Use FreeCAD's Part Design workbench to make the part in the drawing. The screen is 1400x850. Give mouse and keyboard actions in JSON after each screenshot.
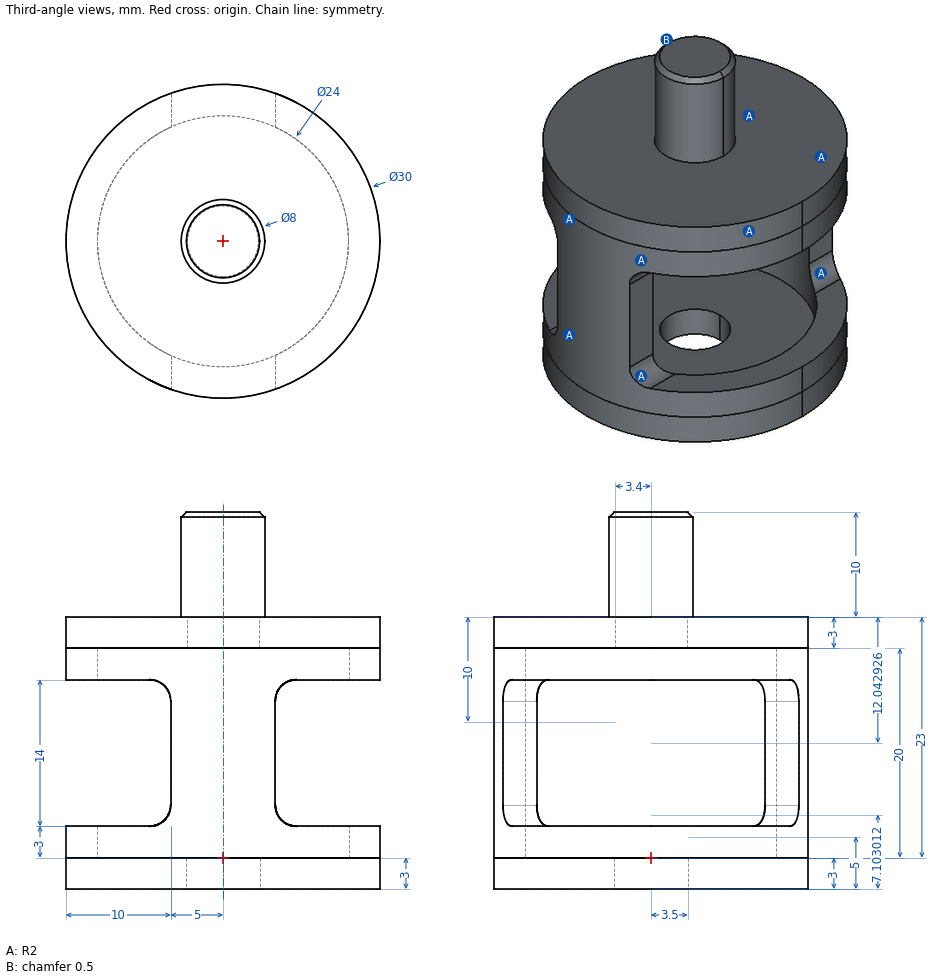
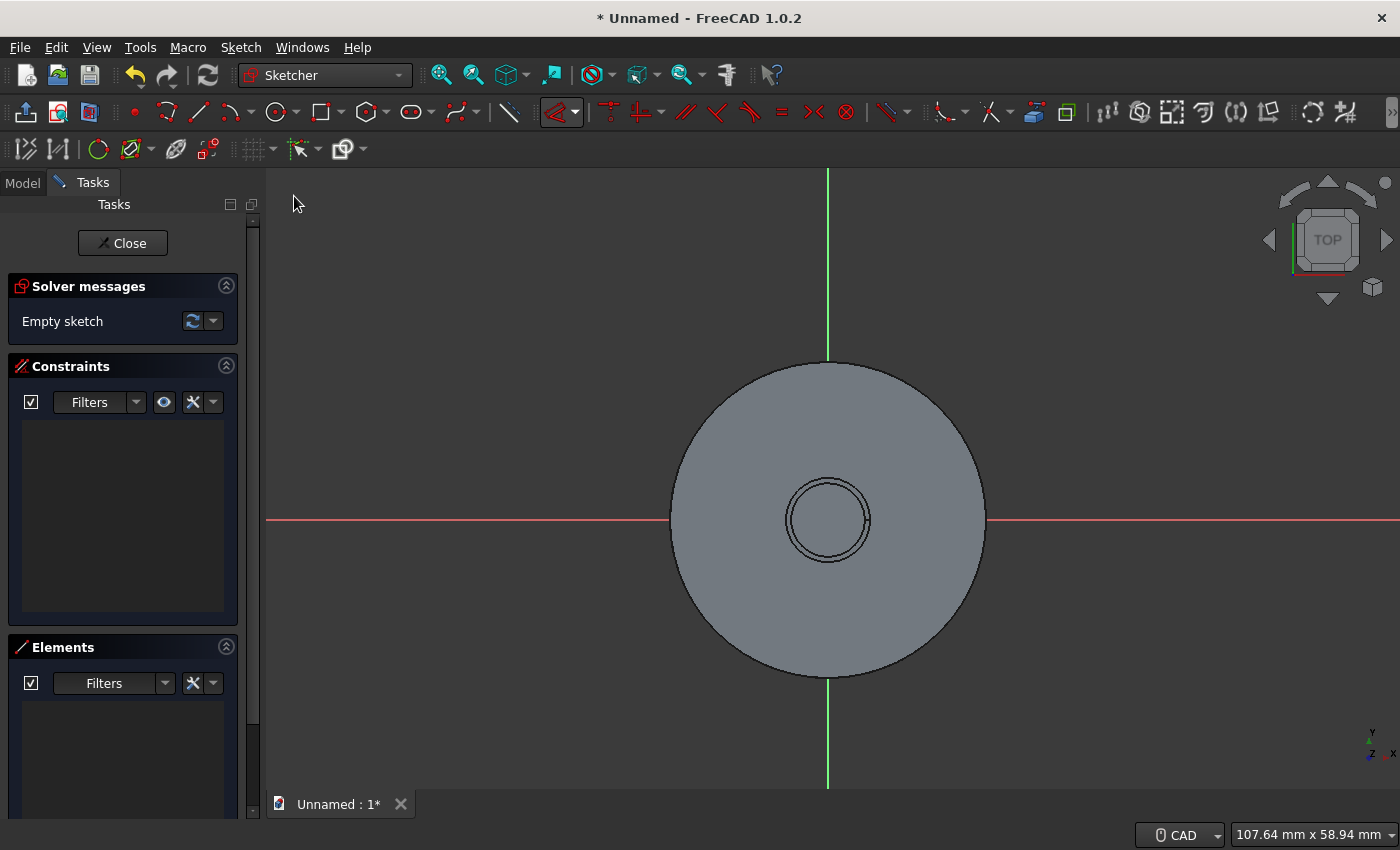
{"action": "key", "text": "g c"}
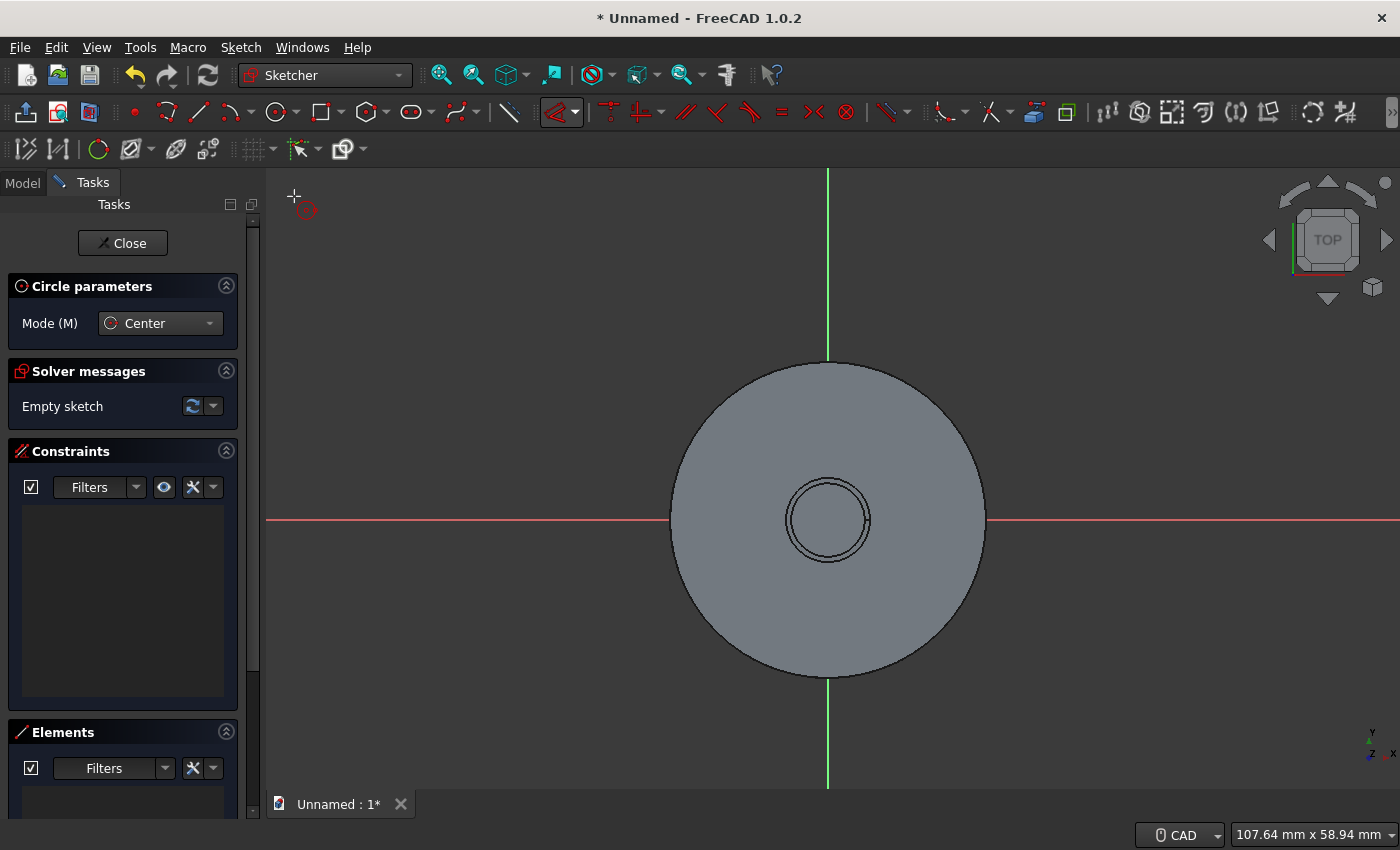
{"action": "left_click", "coordinate": [828, 520]}
{"action": "left_click", "coordinate": [940, 408]}
{"action": "key", "text": "Escape"}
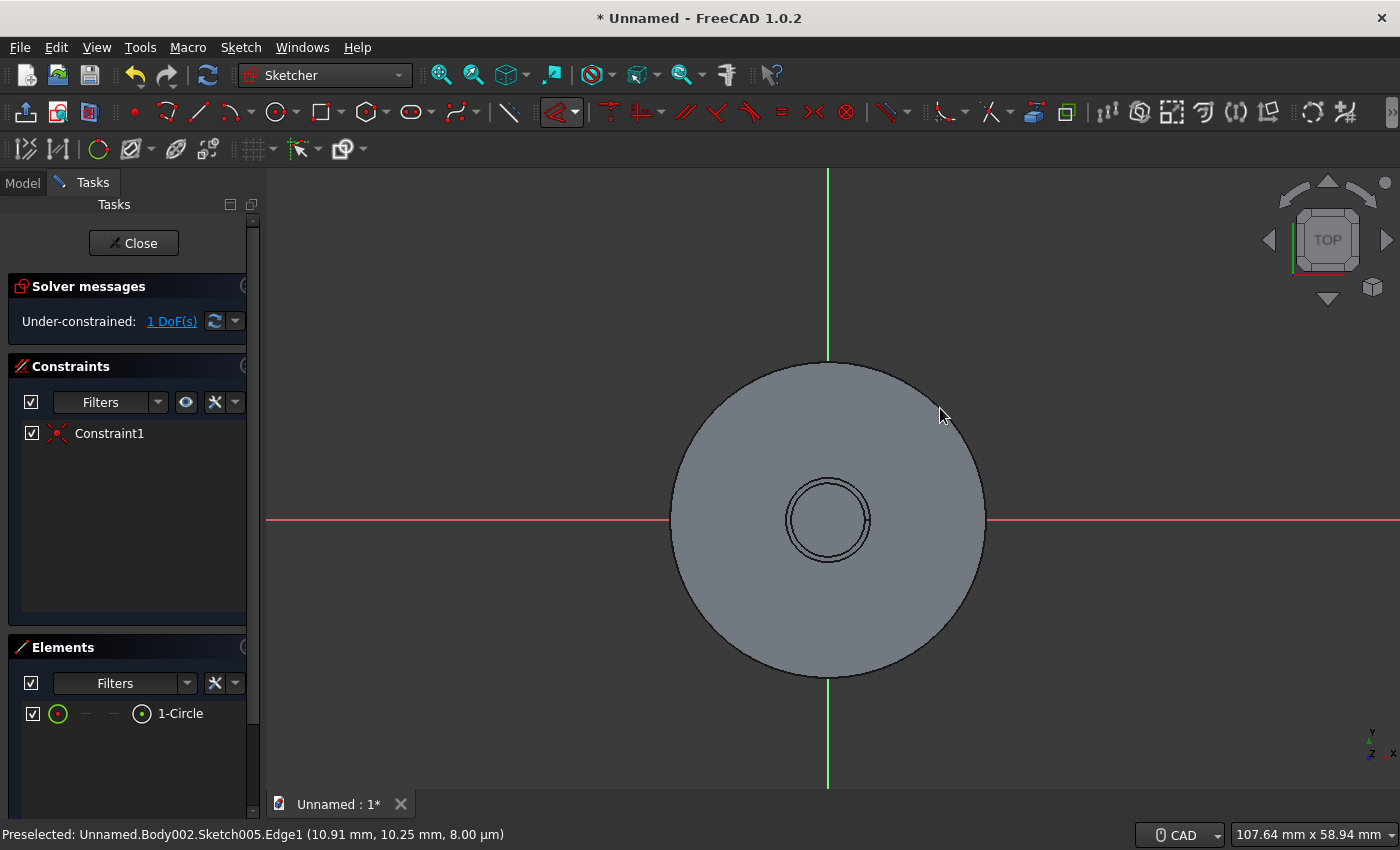
{"action": "left_click", "coordinate": [939, 408]}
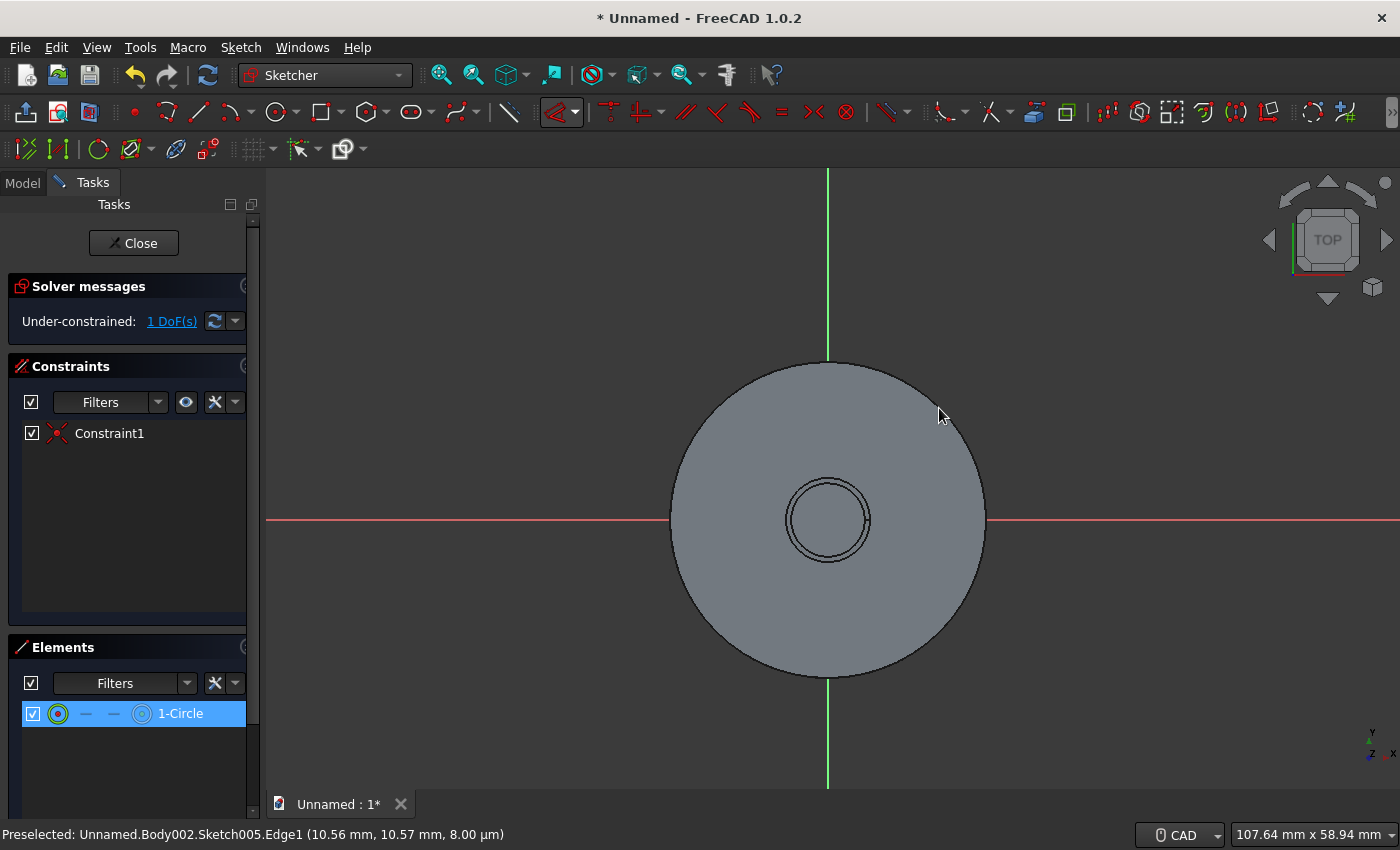
{"action": "left_click", "coordinate": [578, 112]}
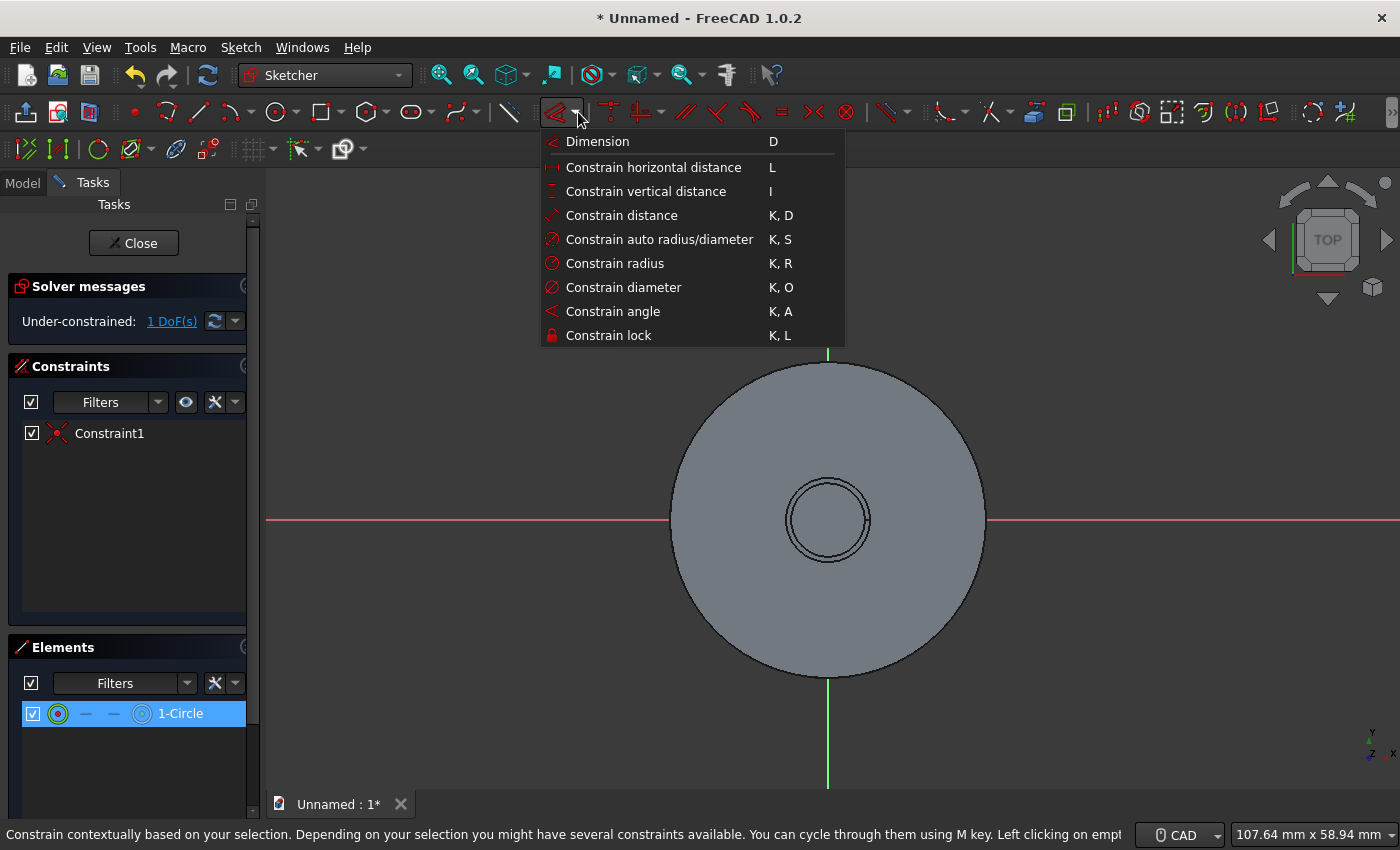
{"action": "left_click", "coordinate": [693, 287]}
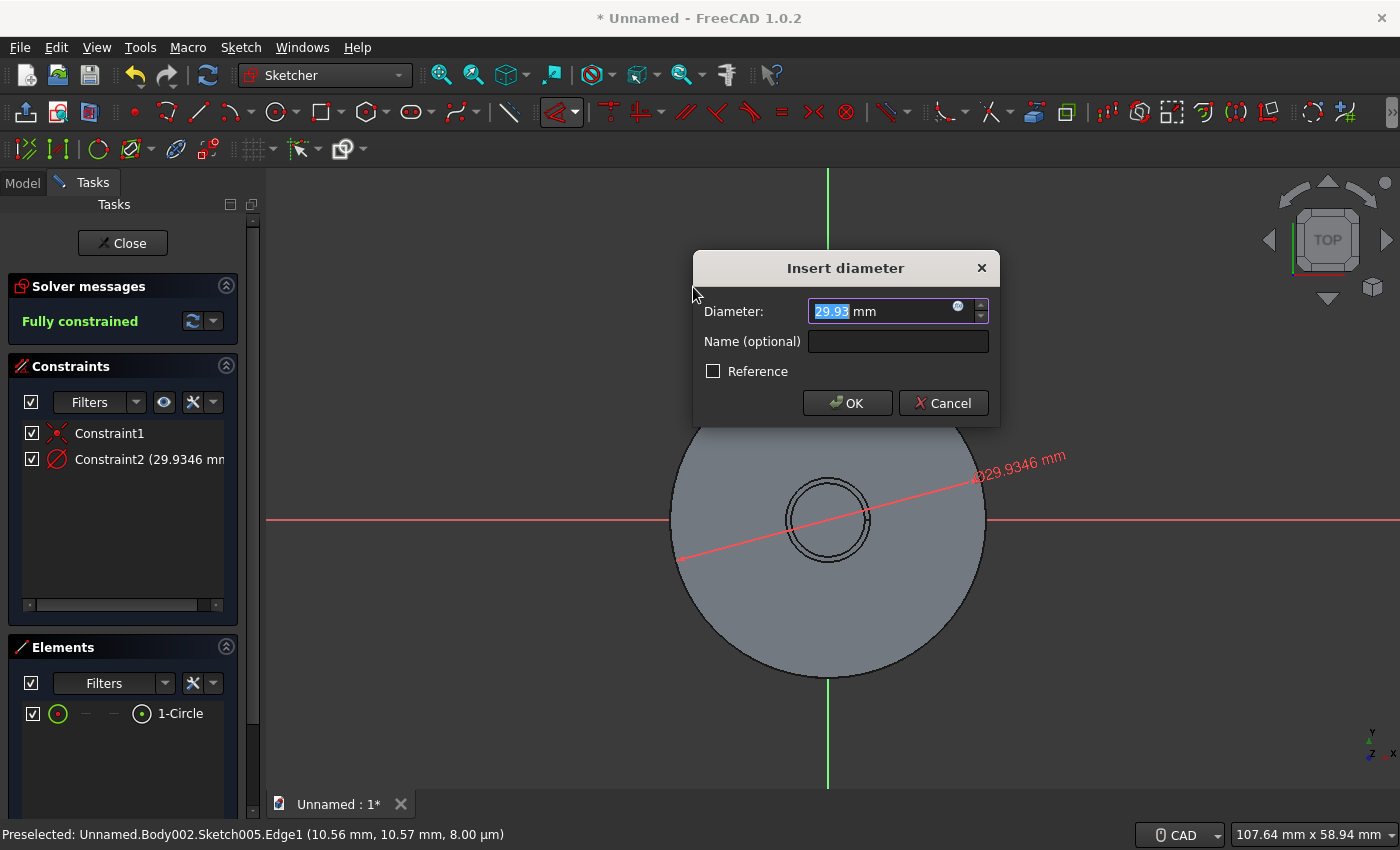
{"action": "type", "text": "30"}
{"action": "key", "text": "Return"}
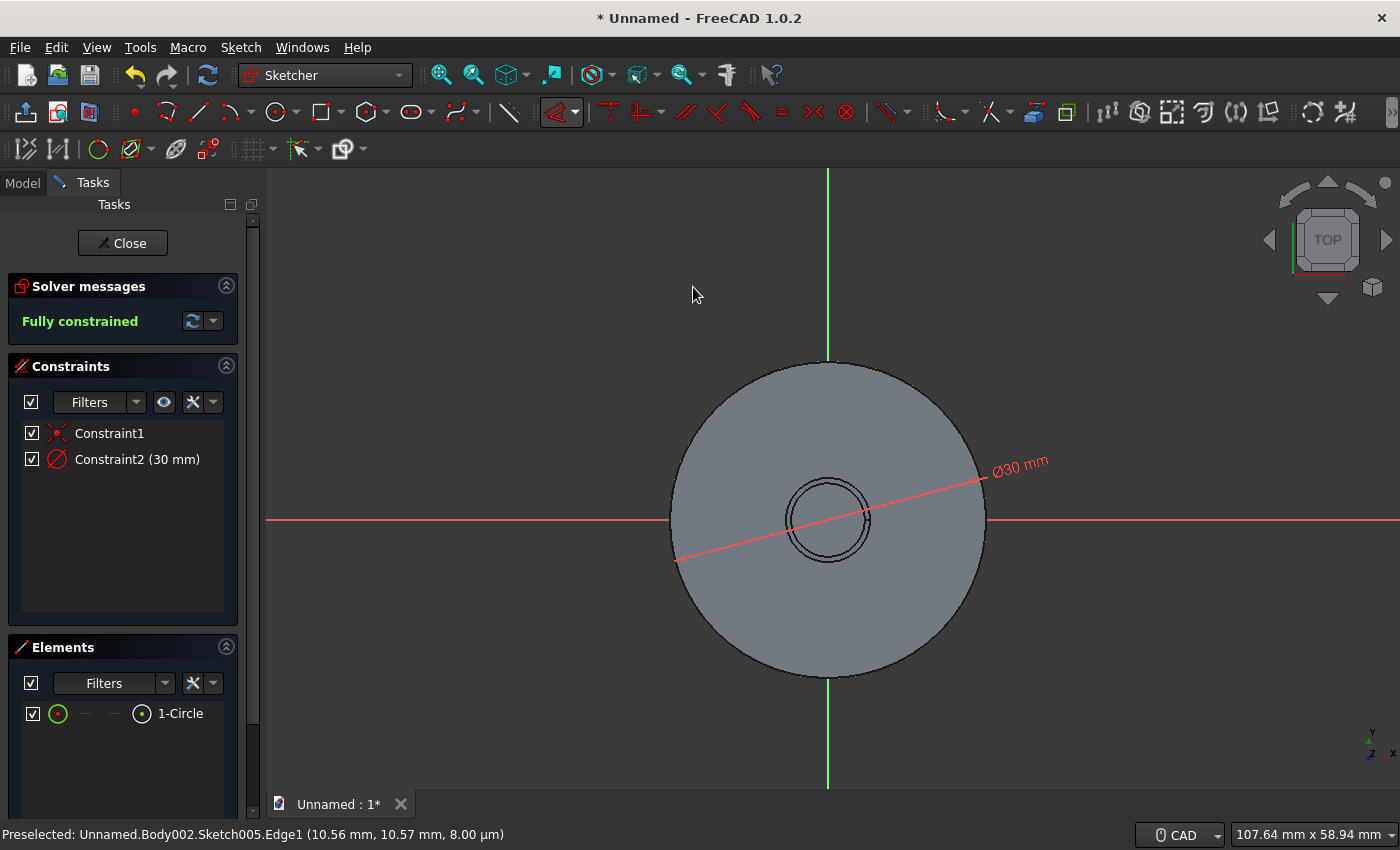
{"action": "left_click", "coordinate": [123, 243]}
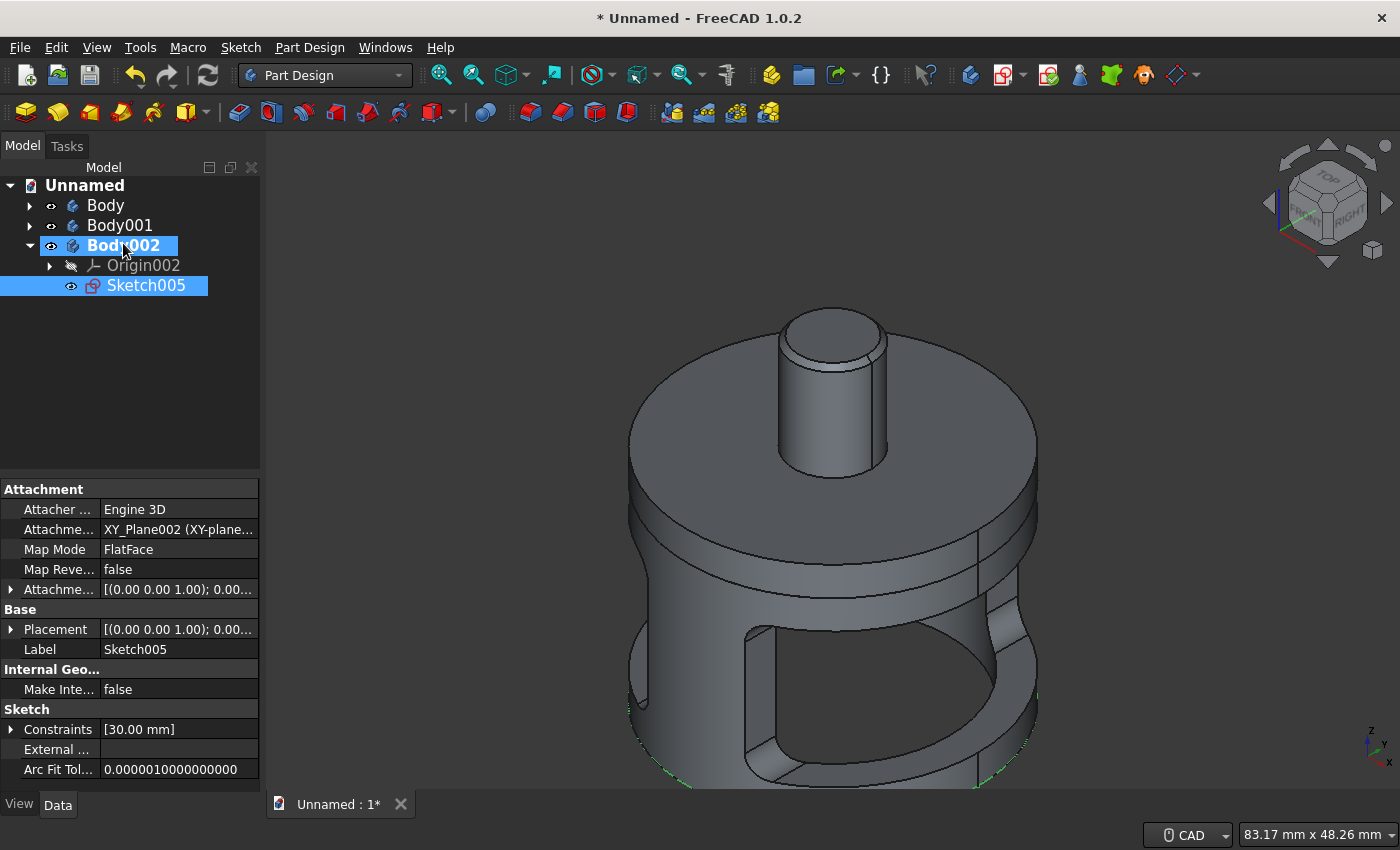
{"action": "left_click", "coordinate": [26, 112]}